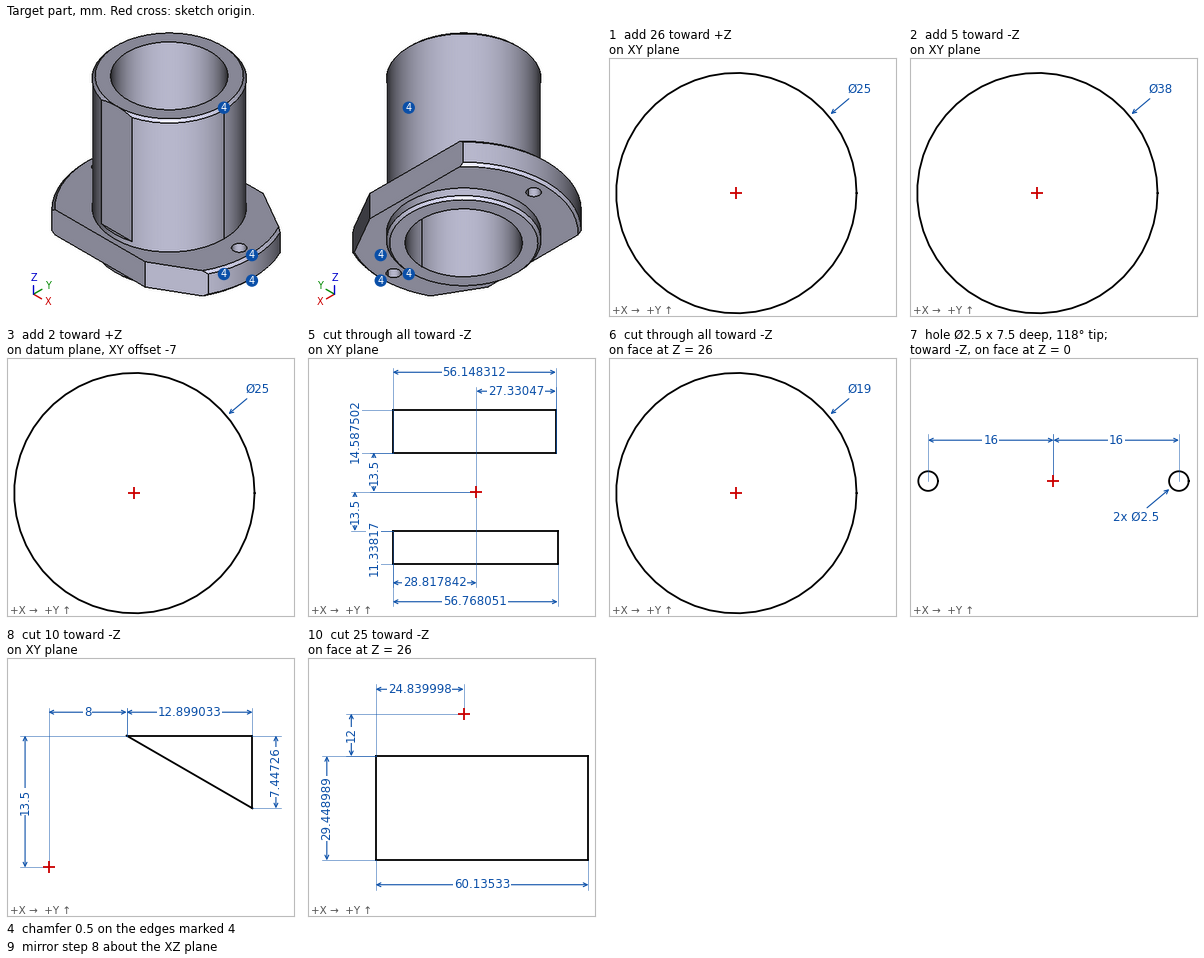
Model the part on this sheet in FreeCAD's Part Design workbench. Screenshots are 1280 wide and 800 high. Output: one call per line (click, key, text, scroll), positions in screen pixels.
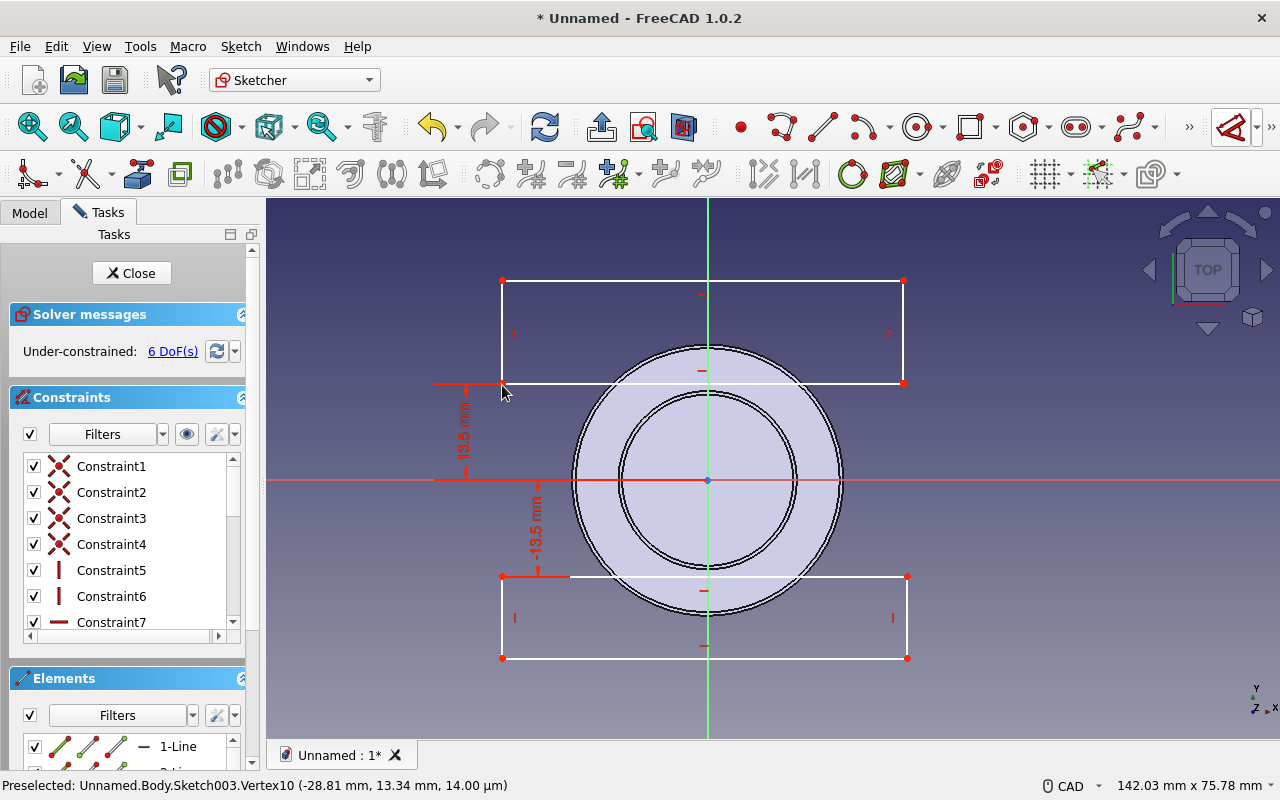
click(502, 601)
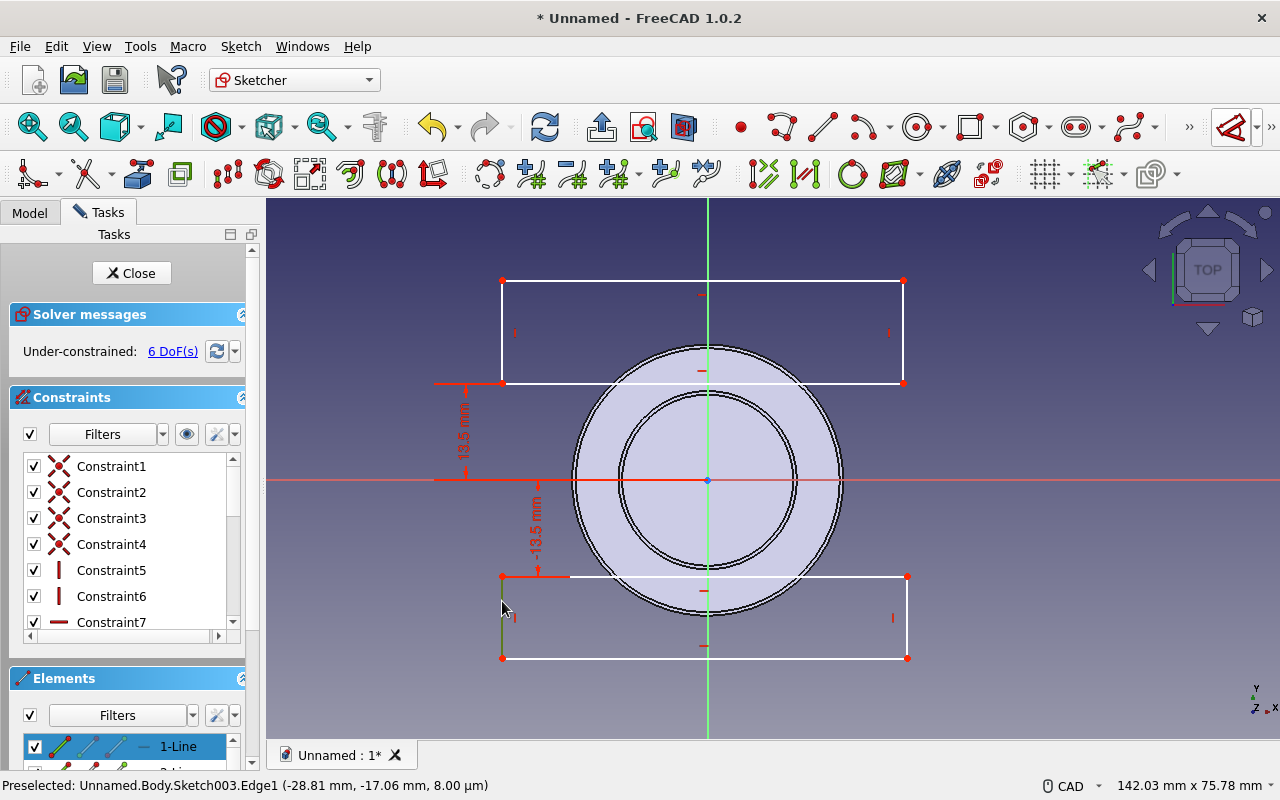
click(1256, 128)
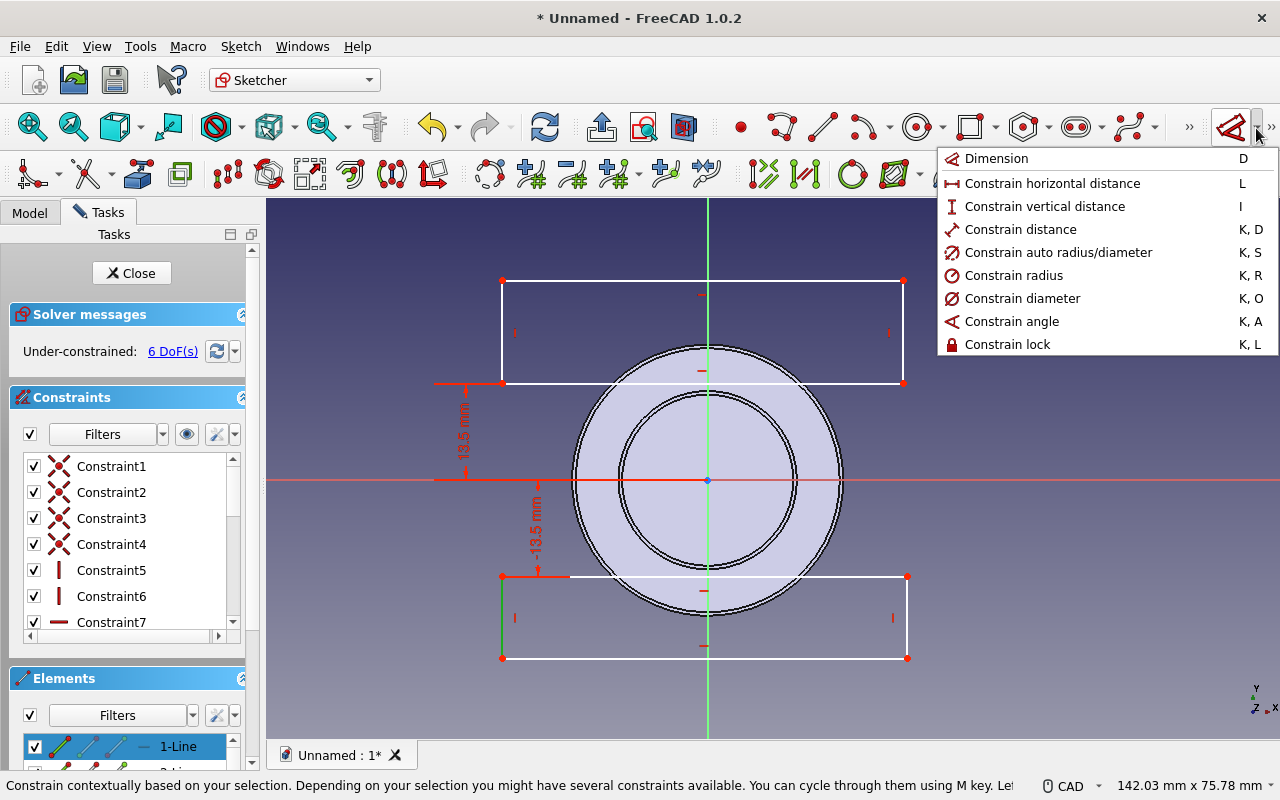
click(1108, 206)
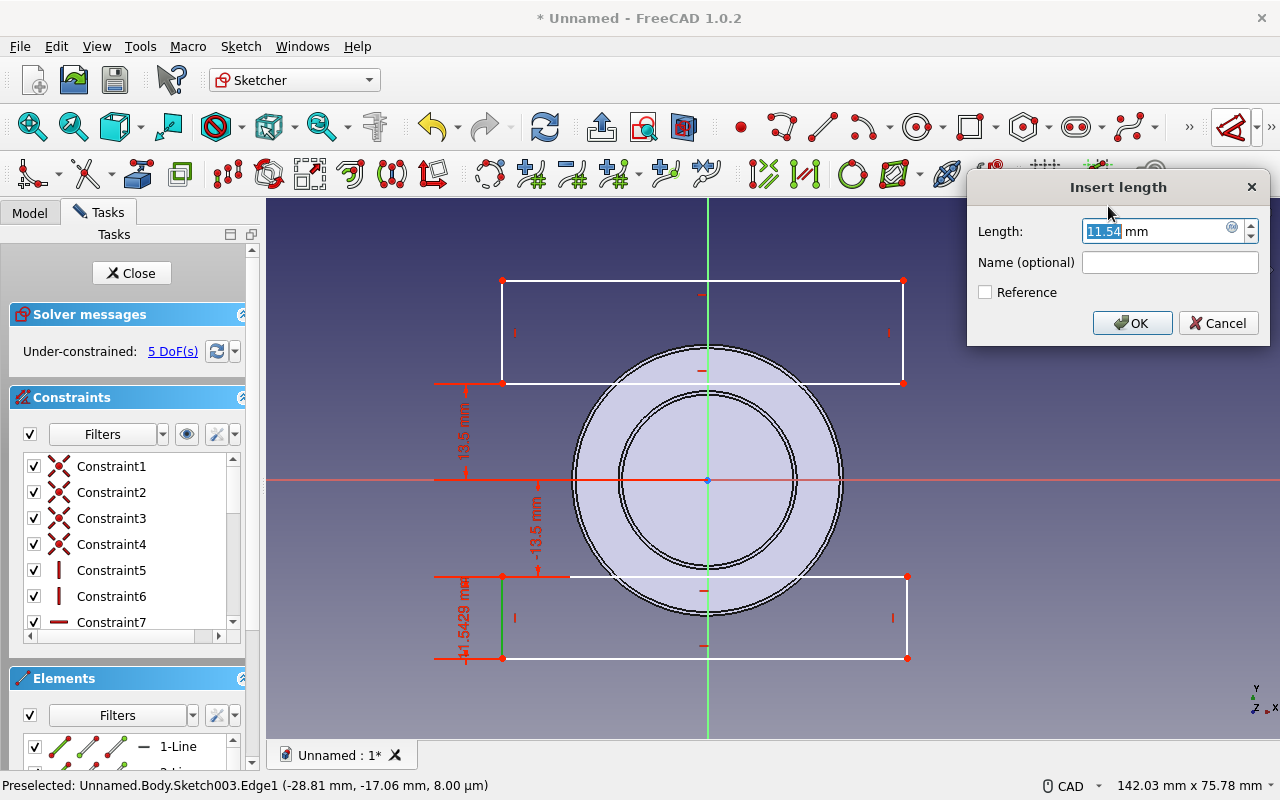
text(11.33817)
key(Return)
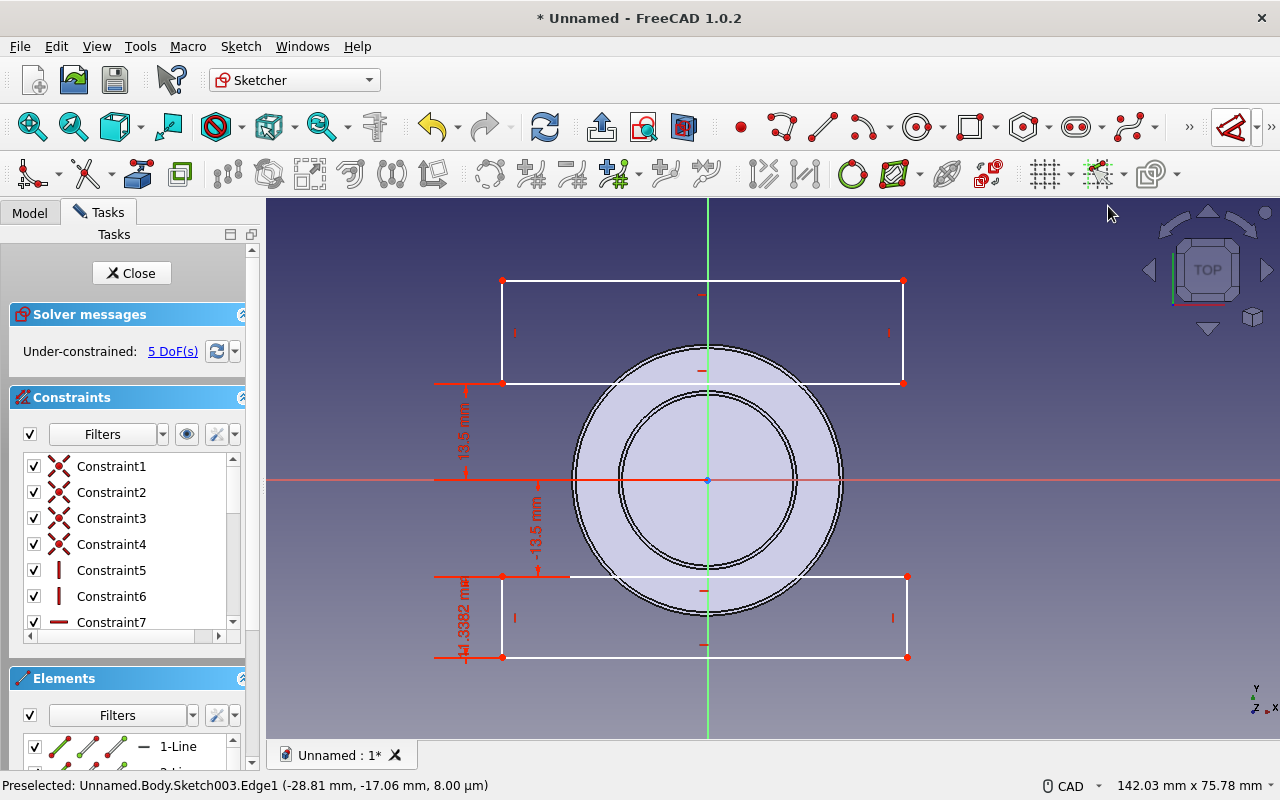
click(624, 658)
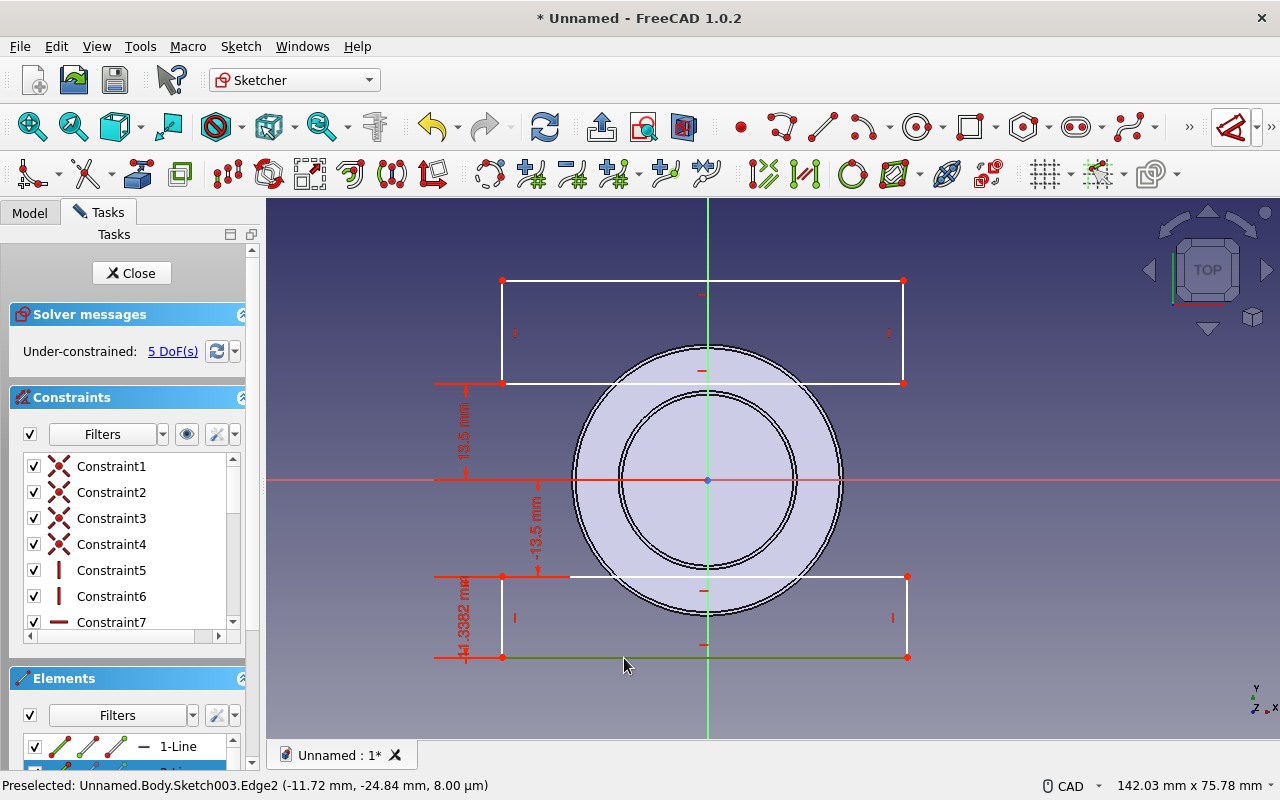
click(1256, 128)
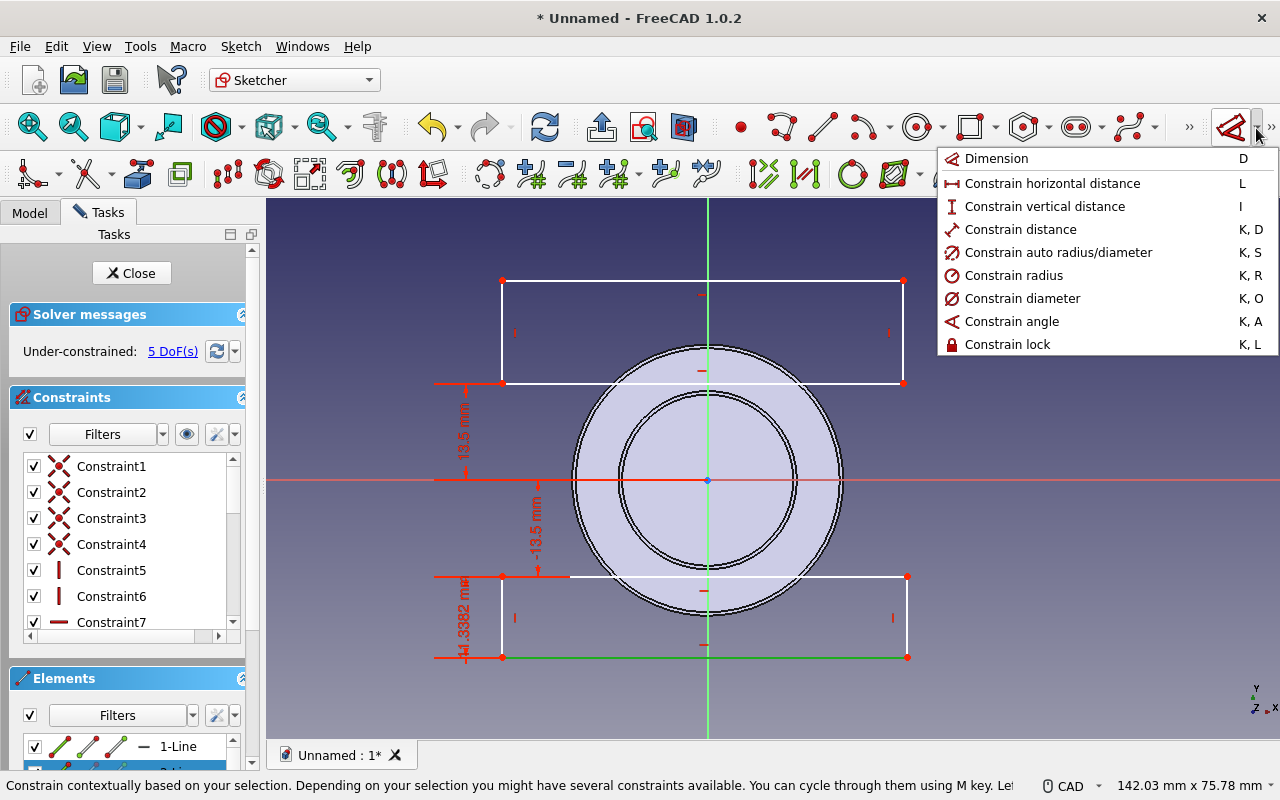
click(1108, 184)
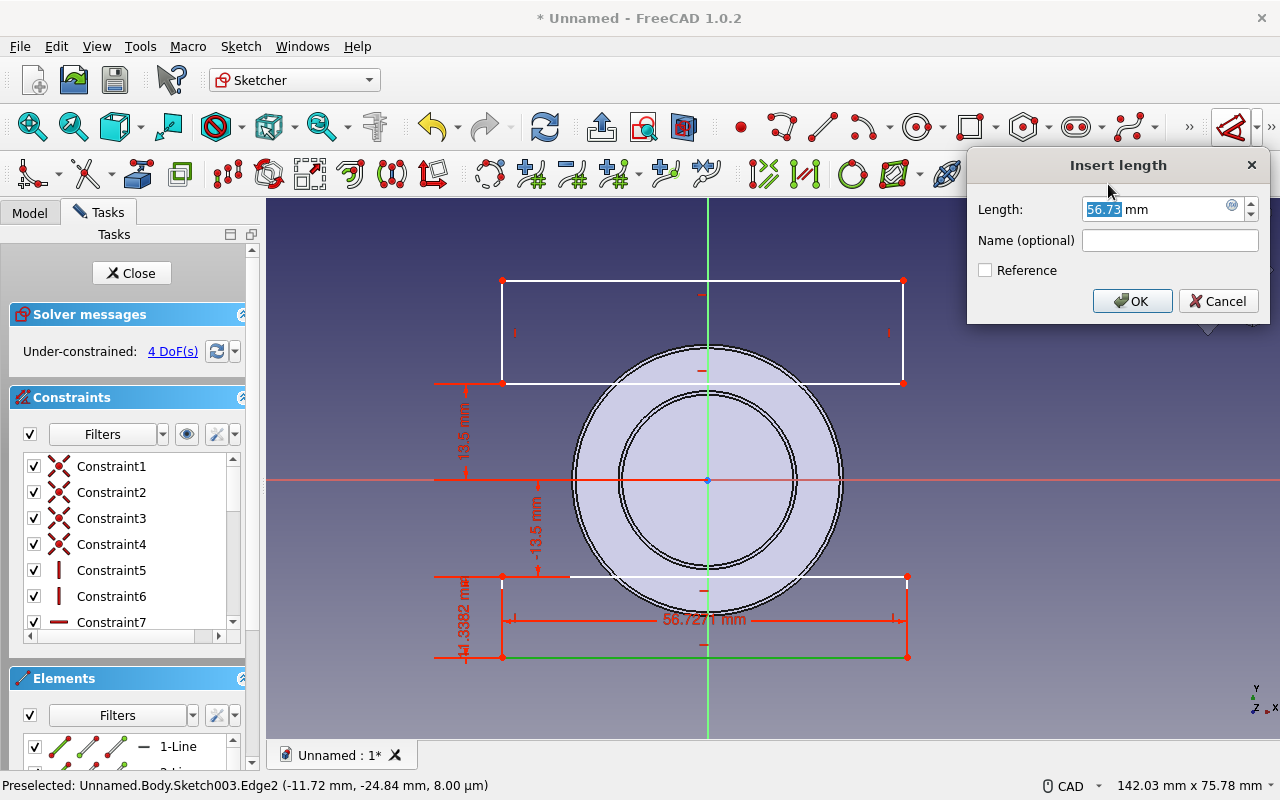
text(56.768051)
key(Return)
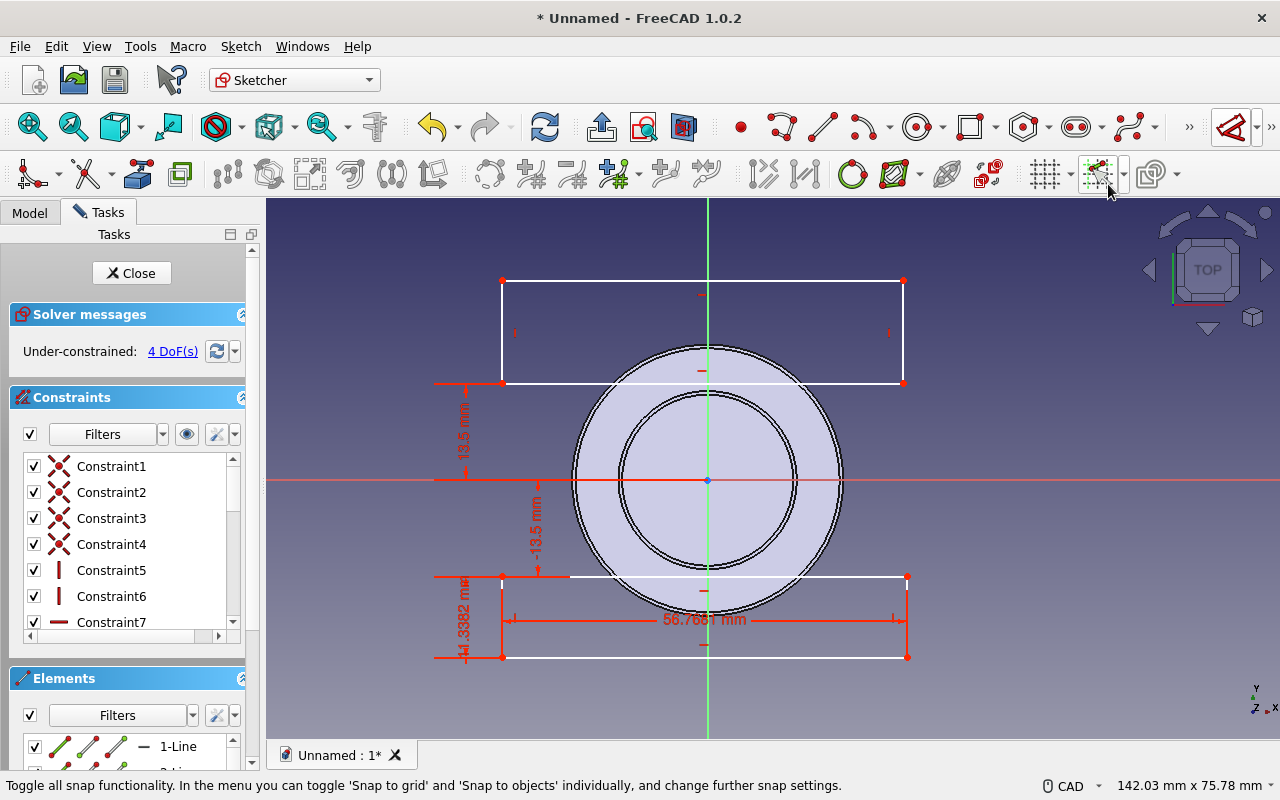
click(502, 312)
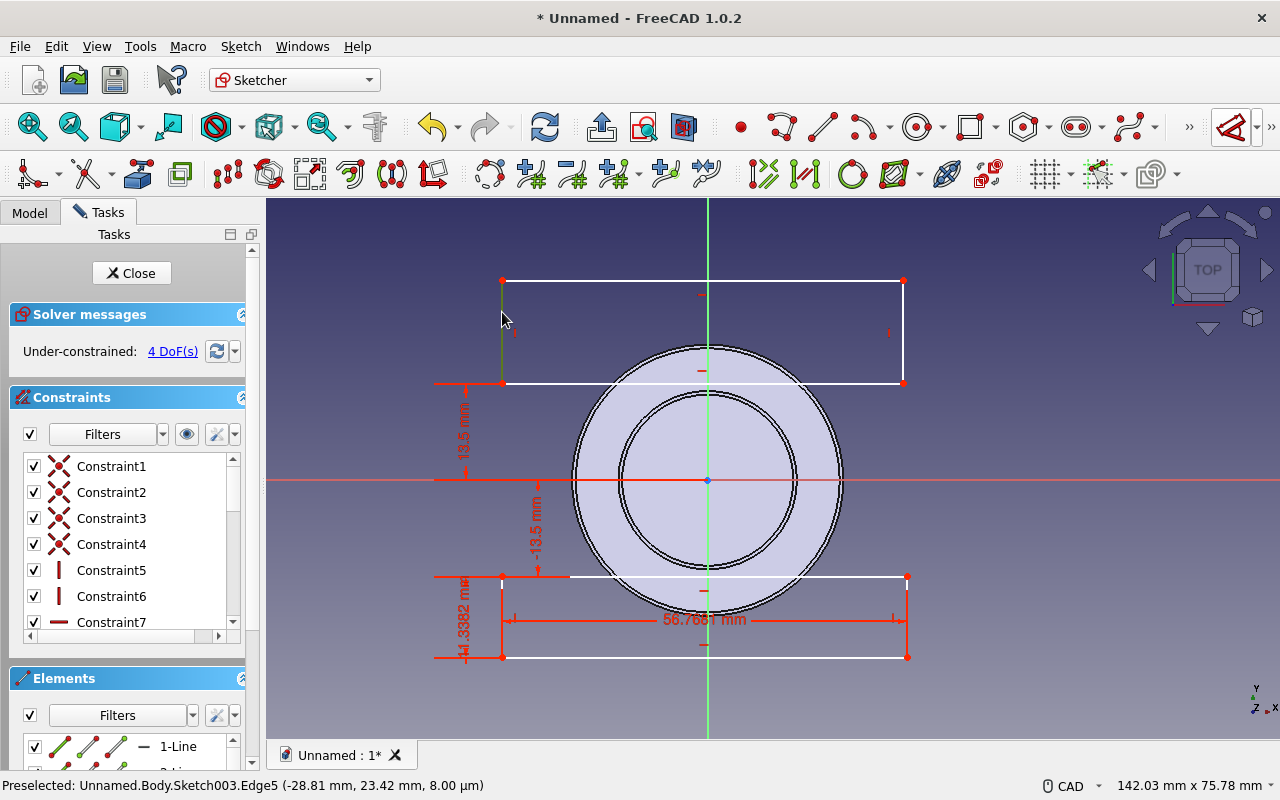
click(1256, 128)